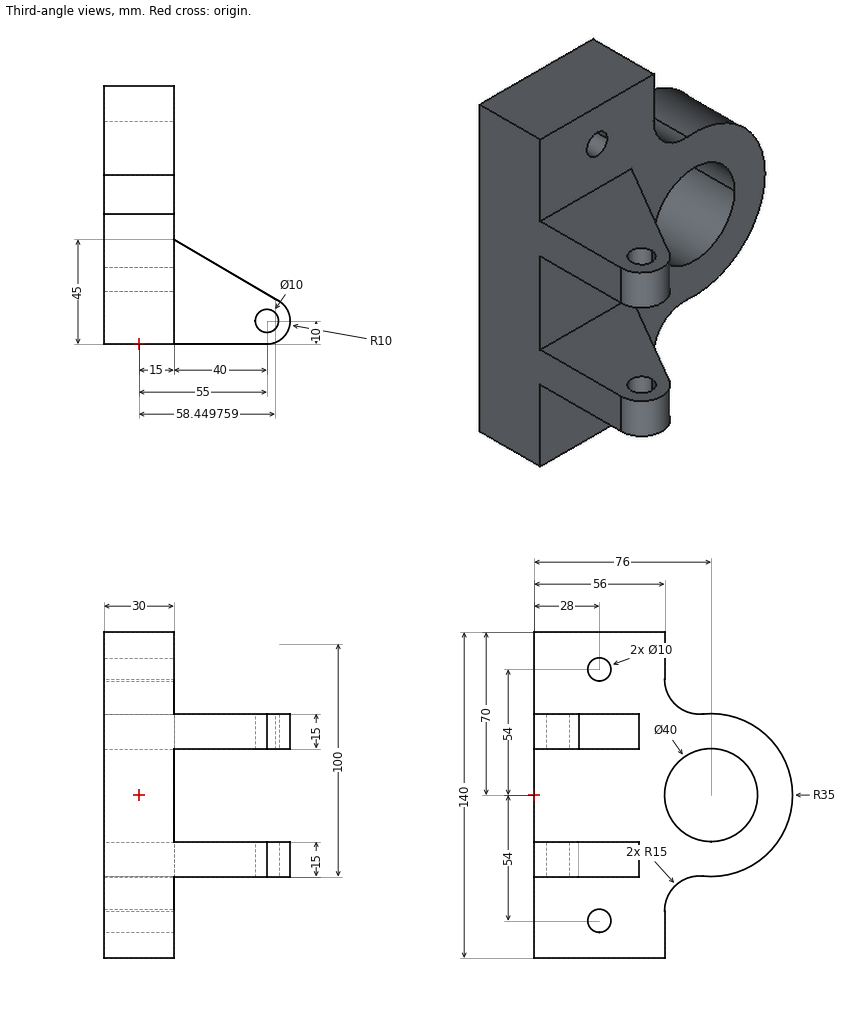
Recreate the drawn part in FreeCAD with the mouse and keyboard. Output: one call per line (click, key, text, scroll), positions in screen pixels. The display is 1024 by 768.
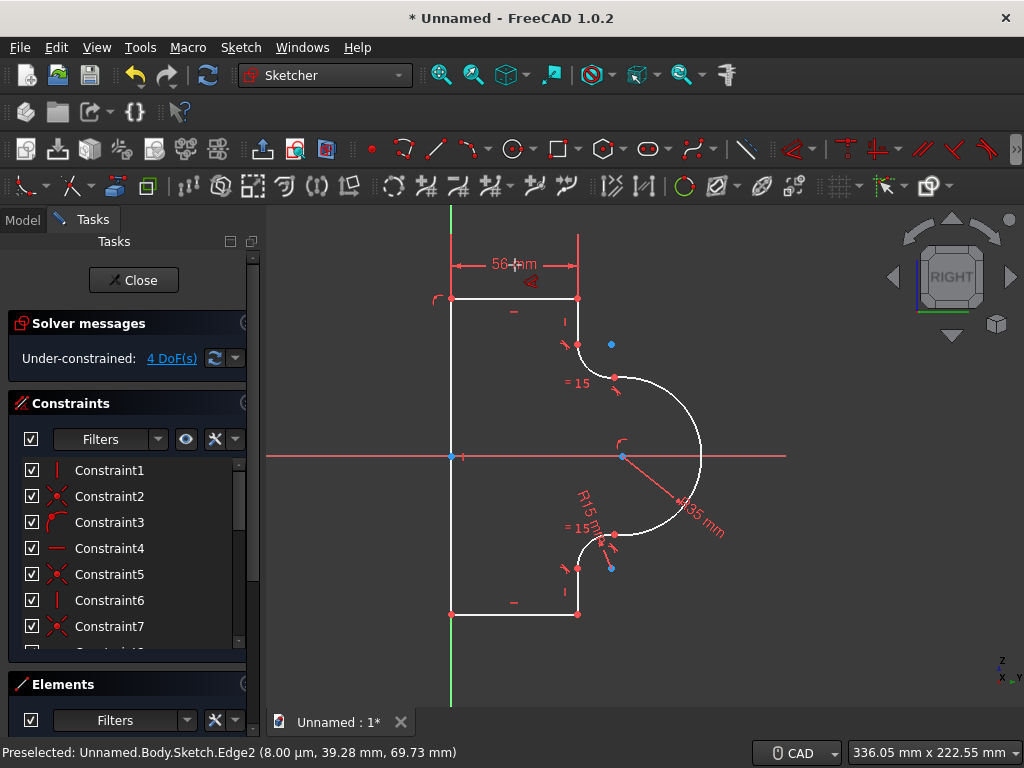
click(489, 615)
click(514, 649)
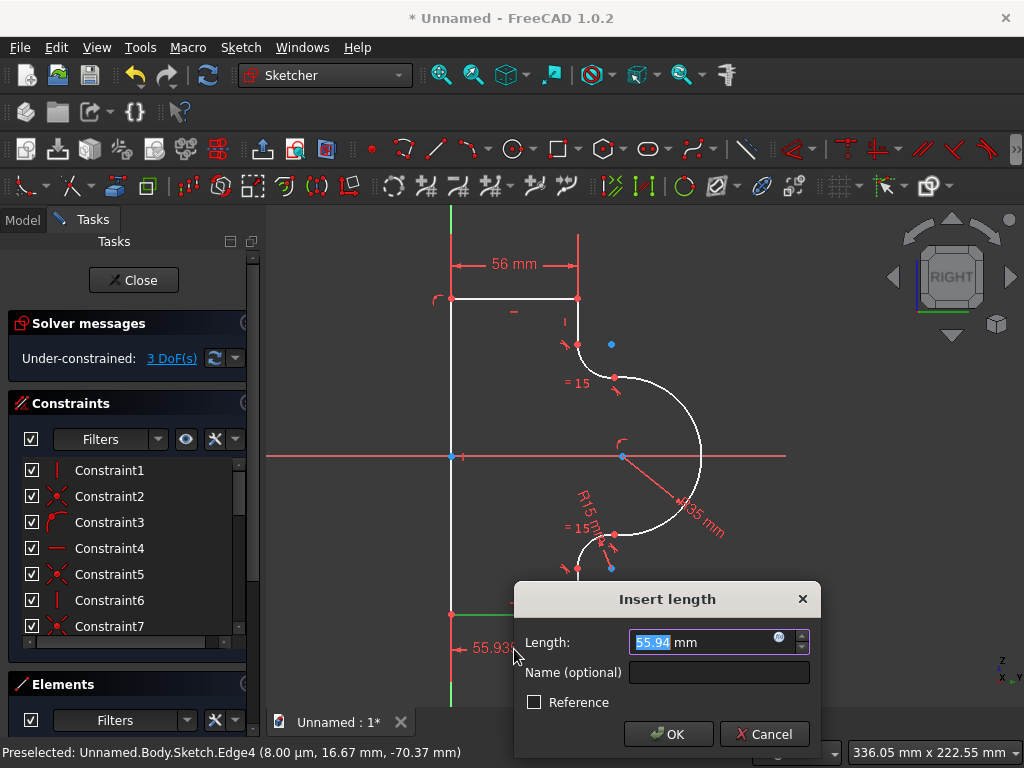
text(56)
key(Return)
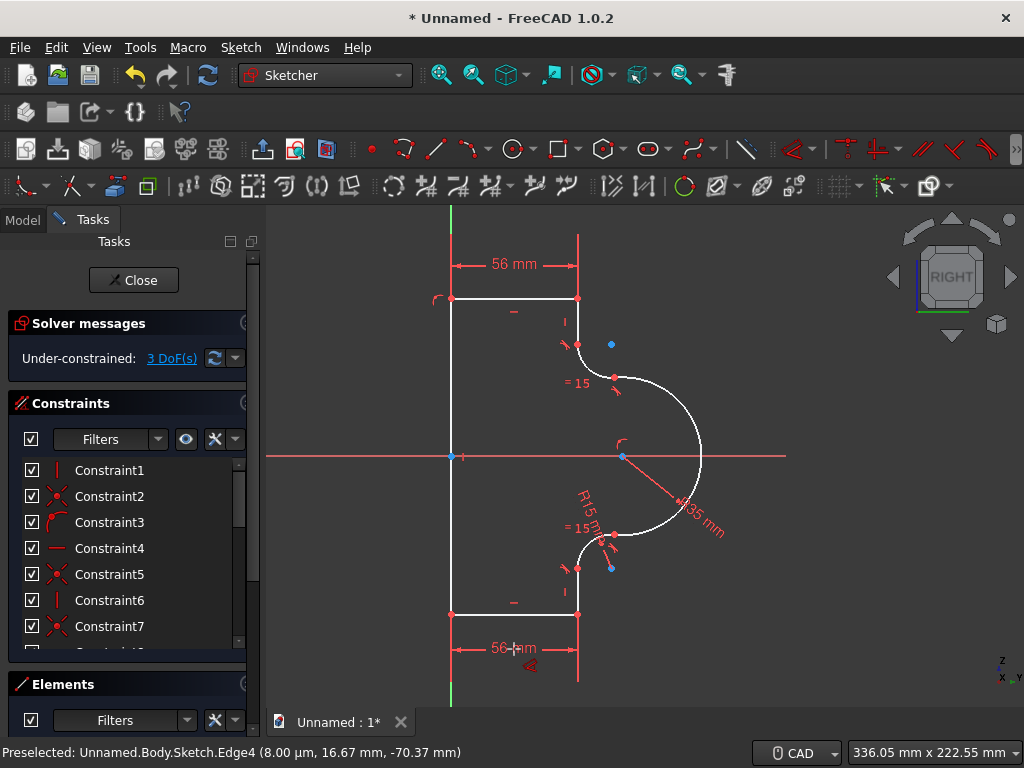
click(451, 394)
click(417, 384)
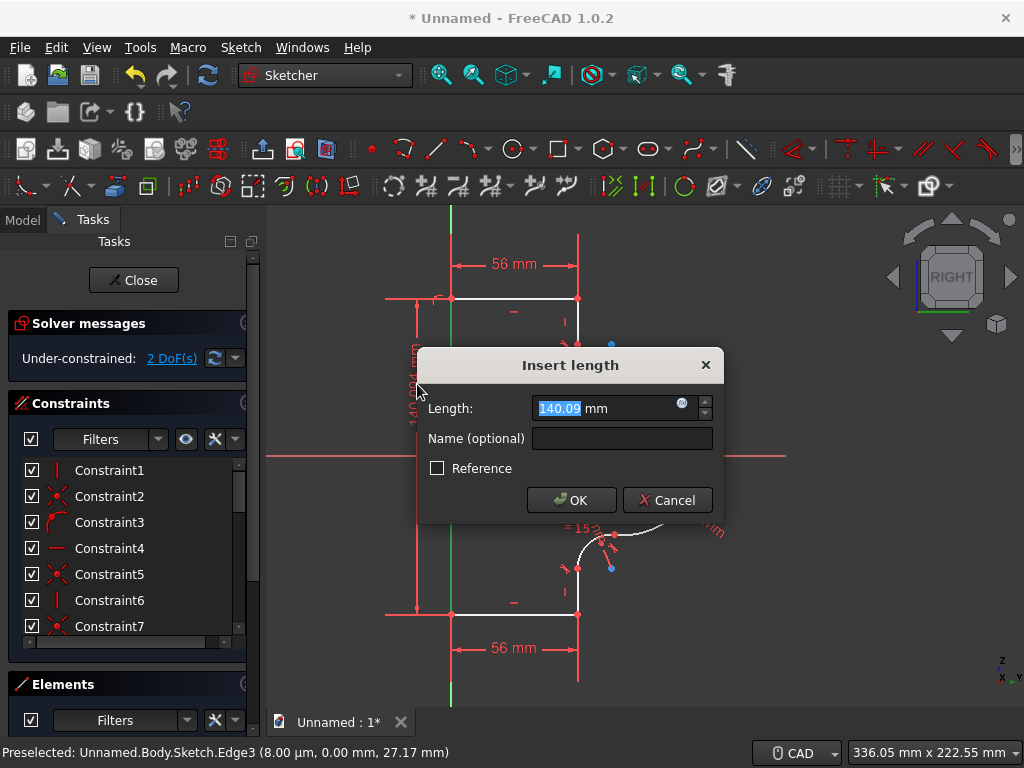
text(140)
key(Return)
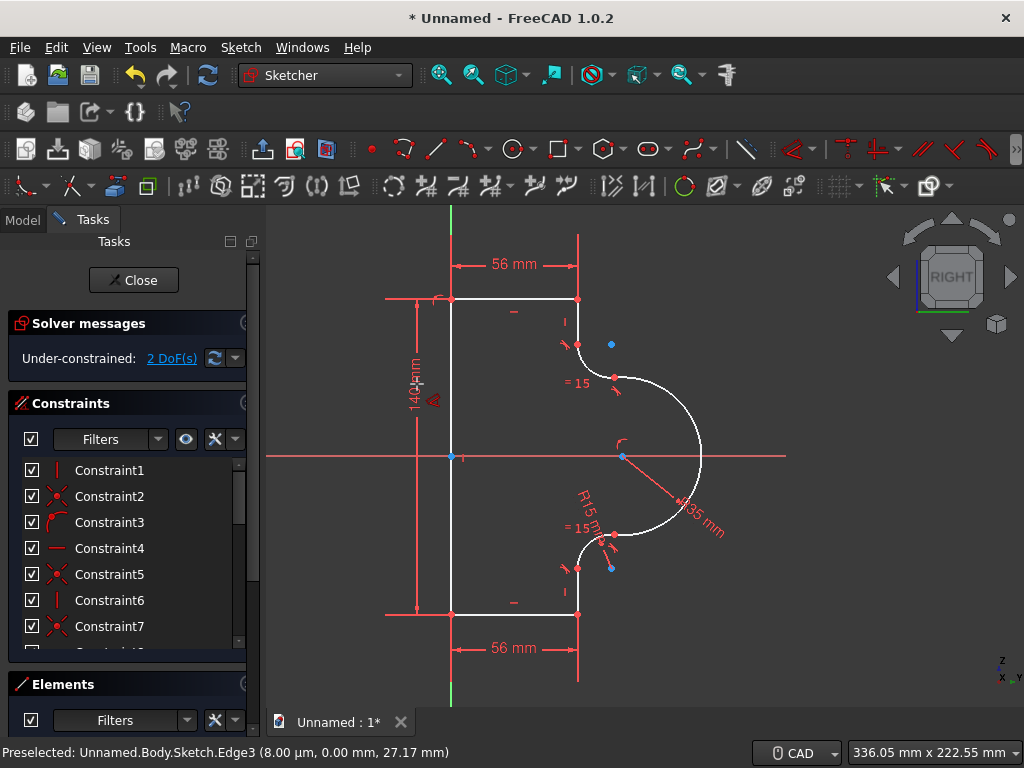
click(578, 299)
click(417, 342)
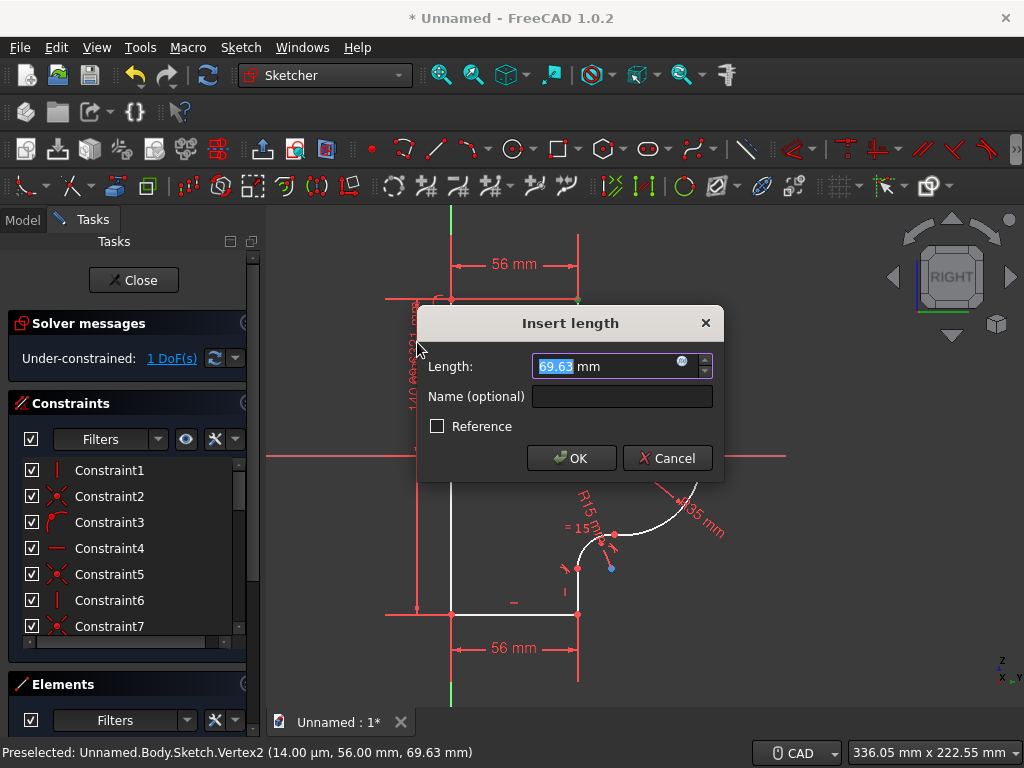
text(70)
key(Return)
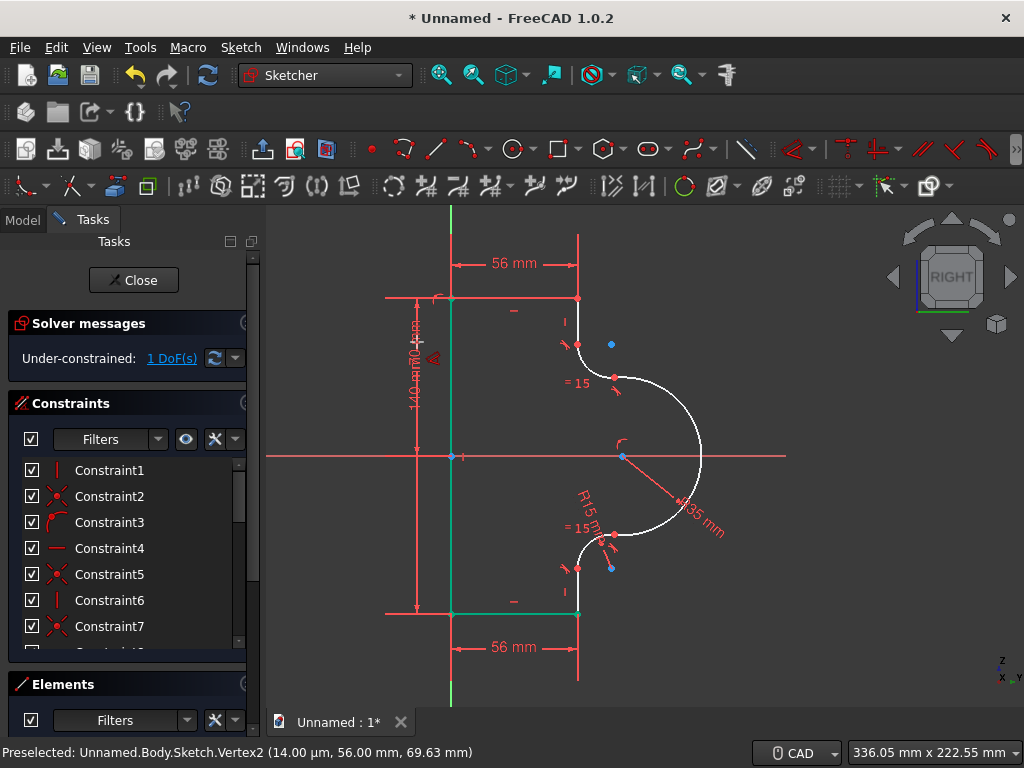
click(622, 456)
click(537, 490)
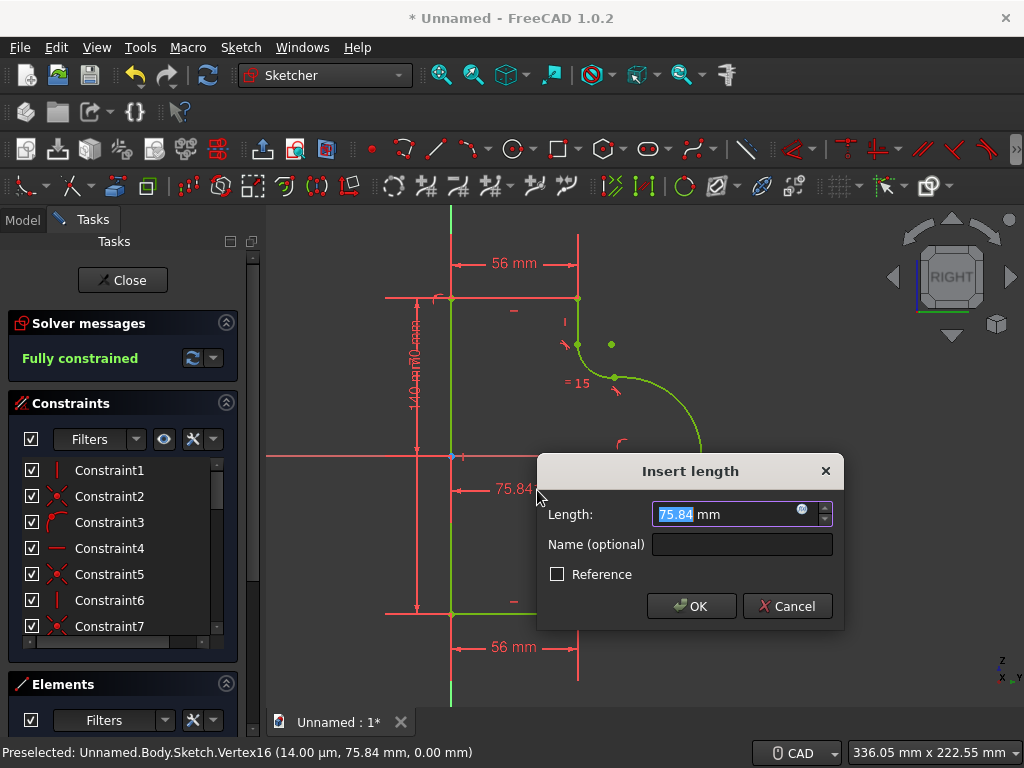
text(76)
key(Return)
key(Escape)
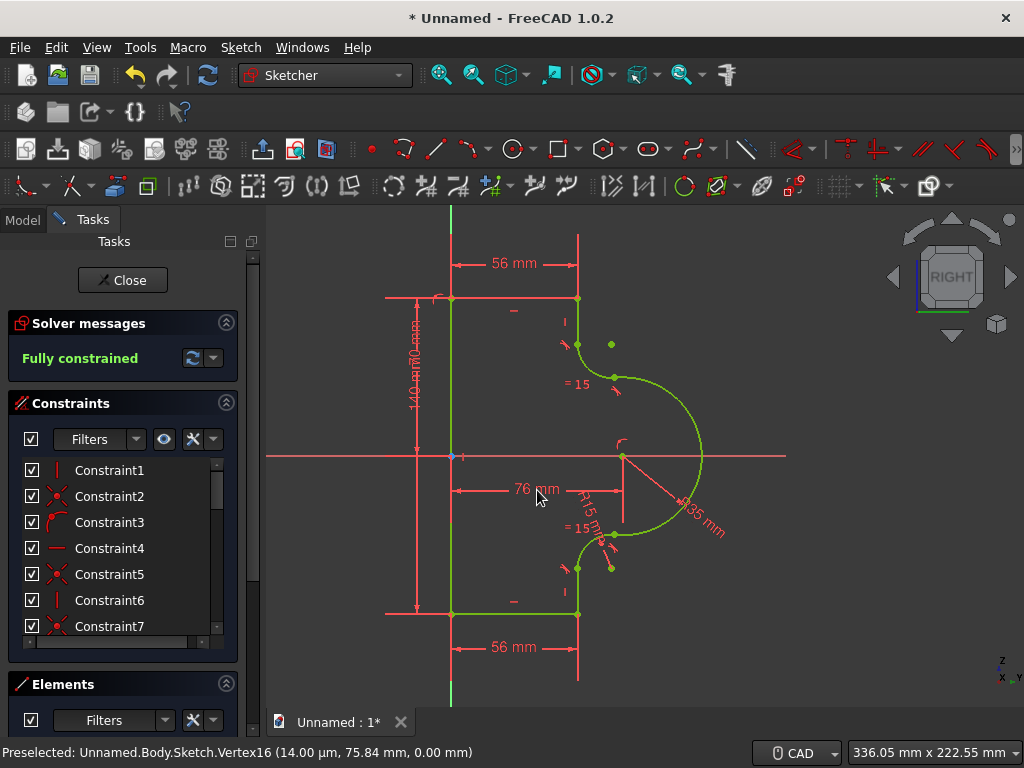
click(123, 280)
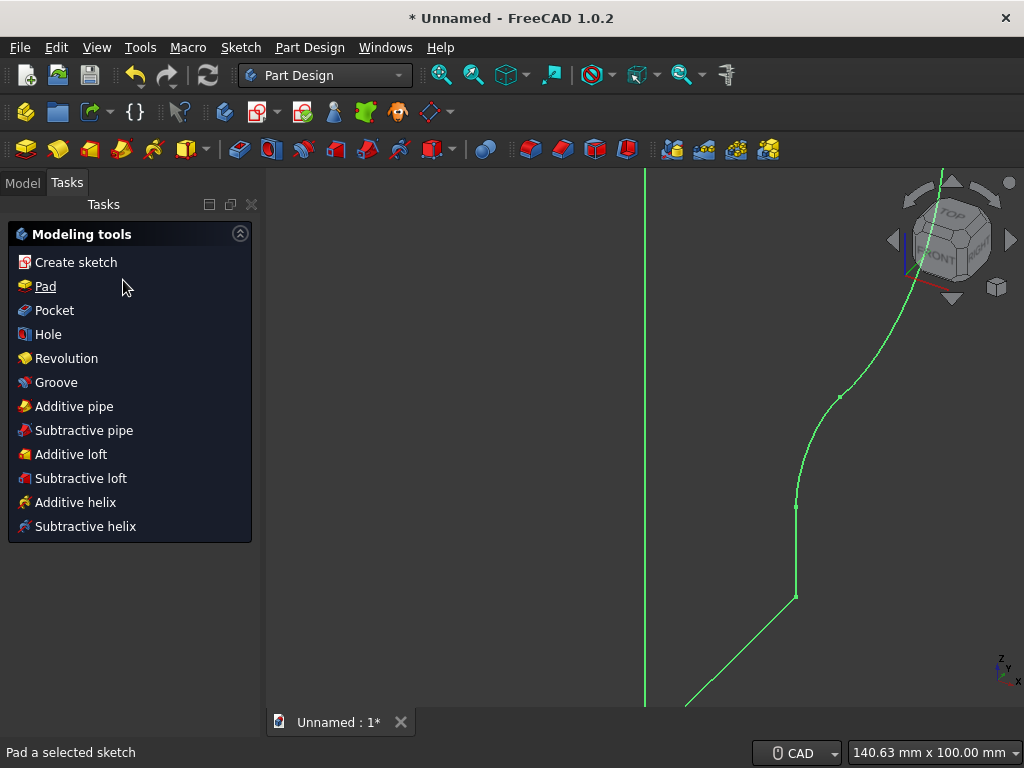
click(26, 150)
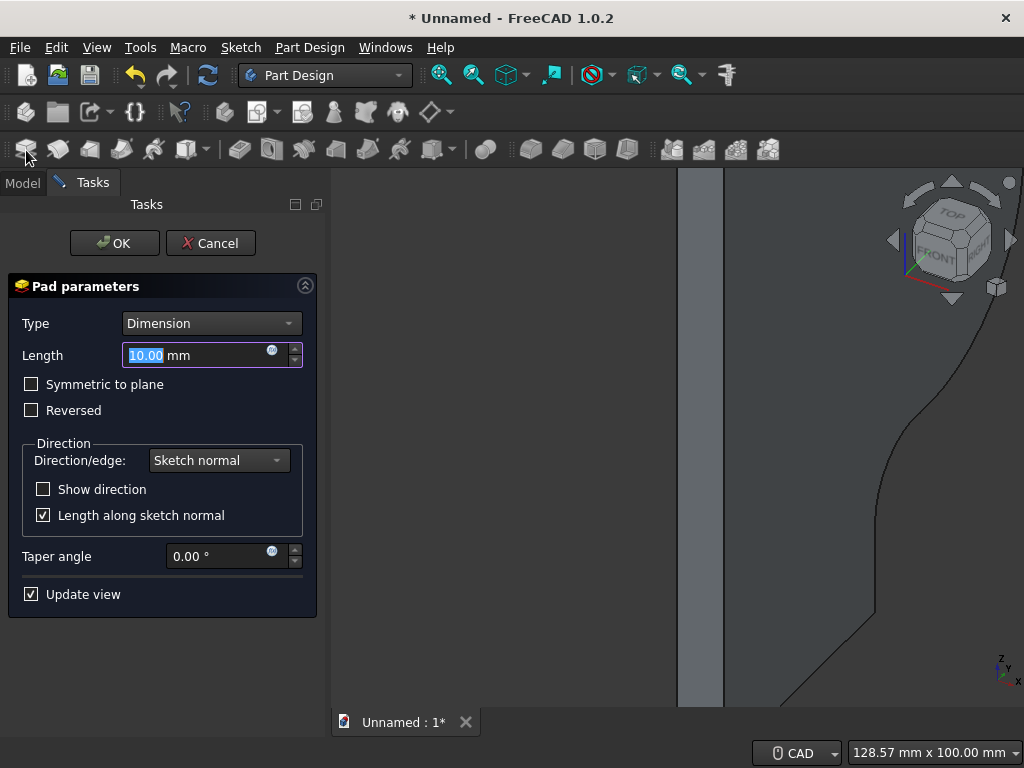
text(30)
key(Tab)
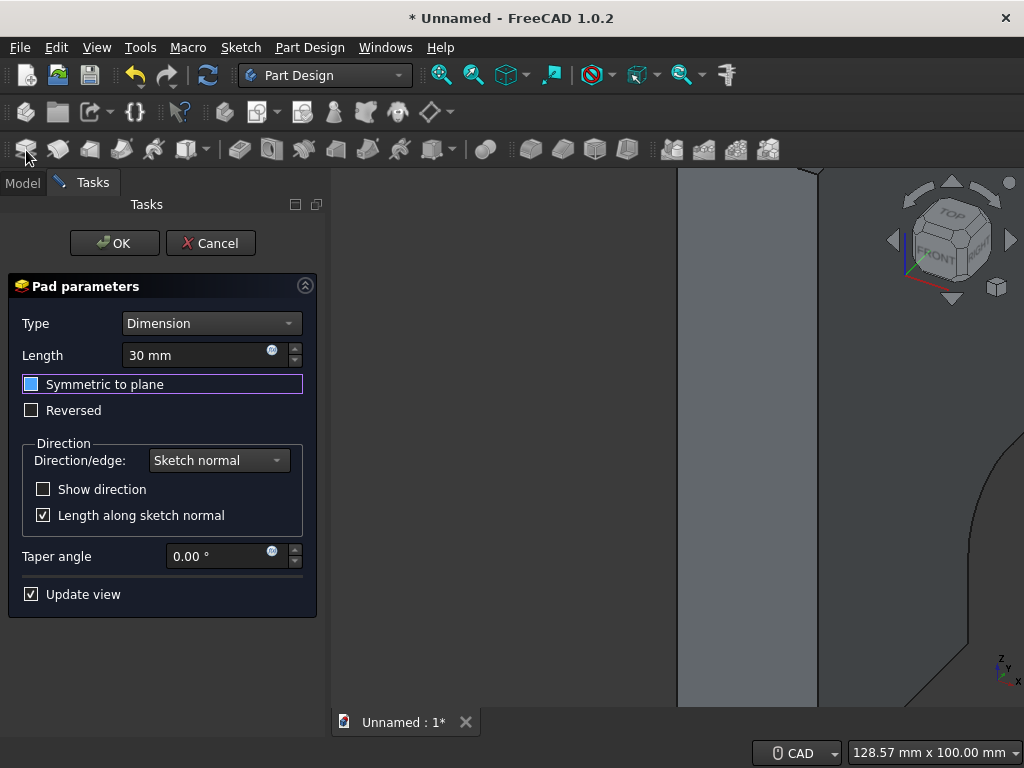
click(30, 384)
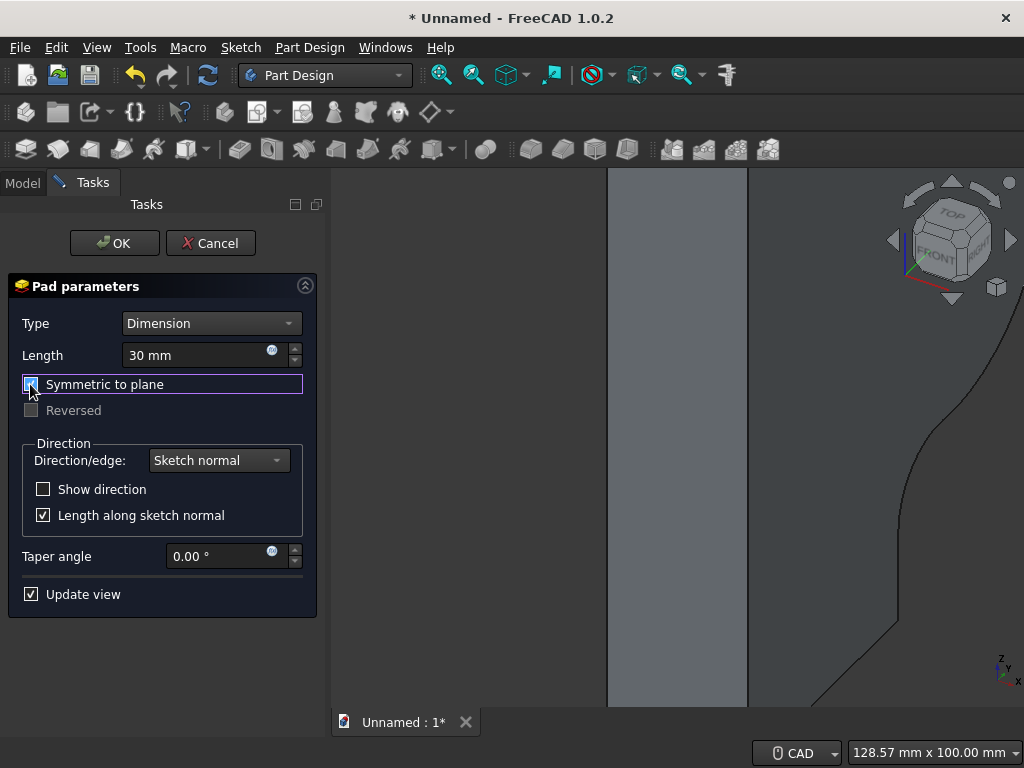
click(115, 243)